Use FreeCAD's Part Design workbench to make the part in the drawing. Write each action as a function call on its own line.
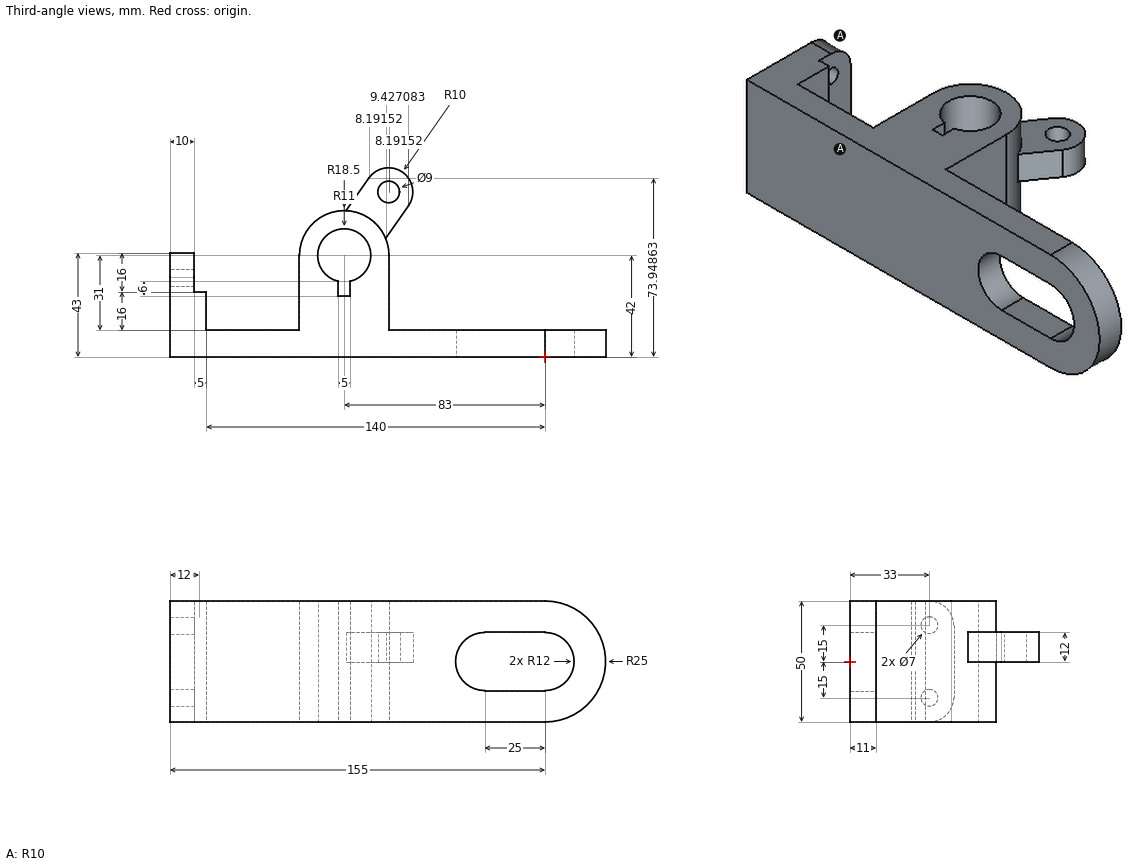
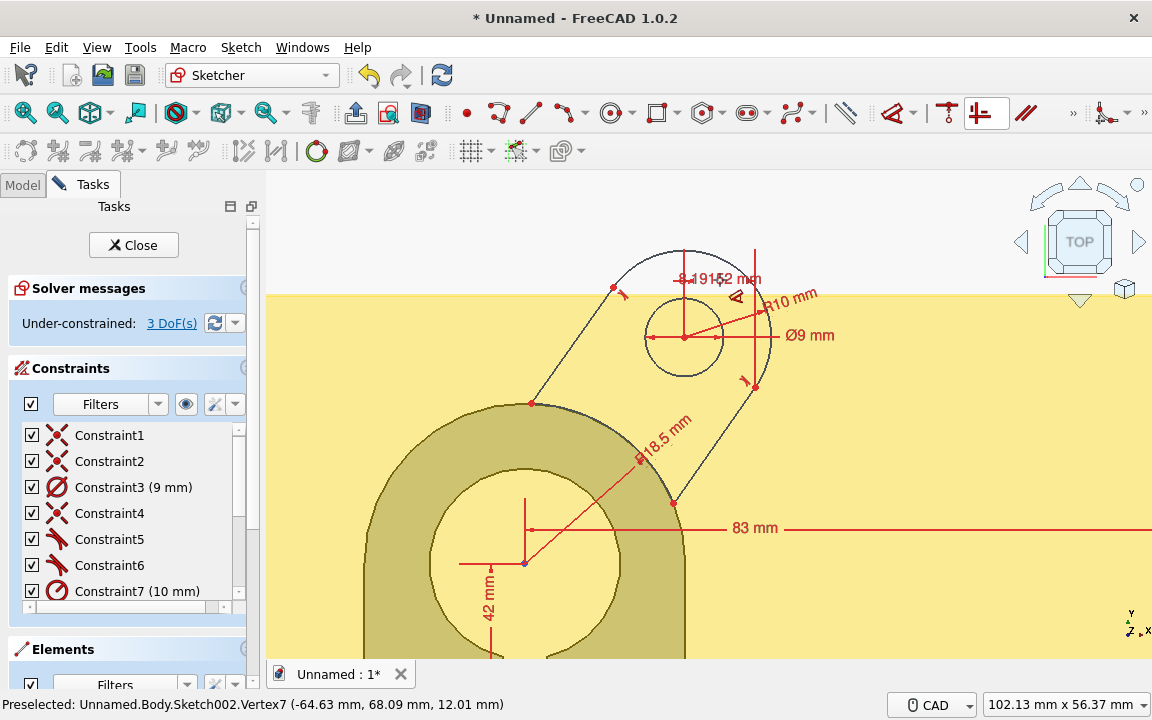
click(614, 287)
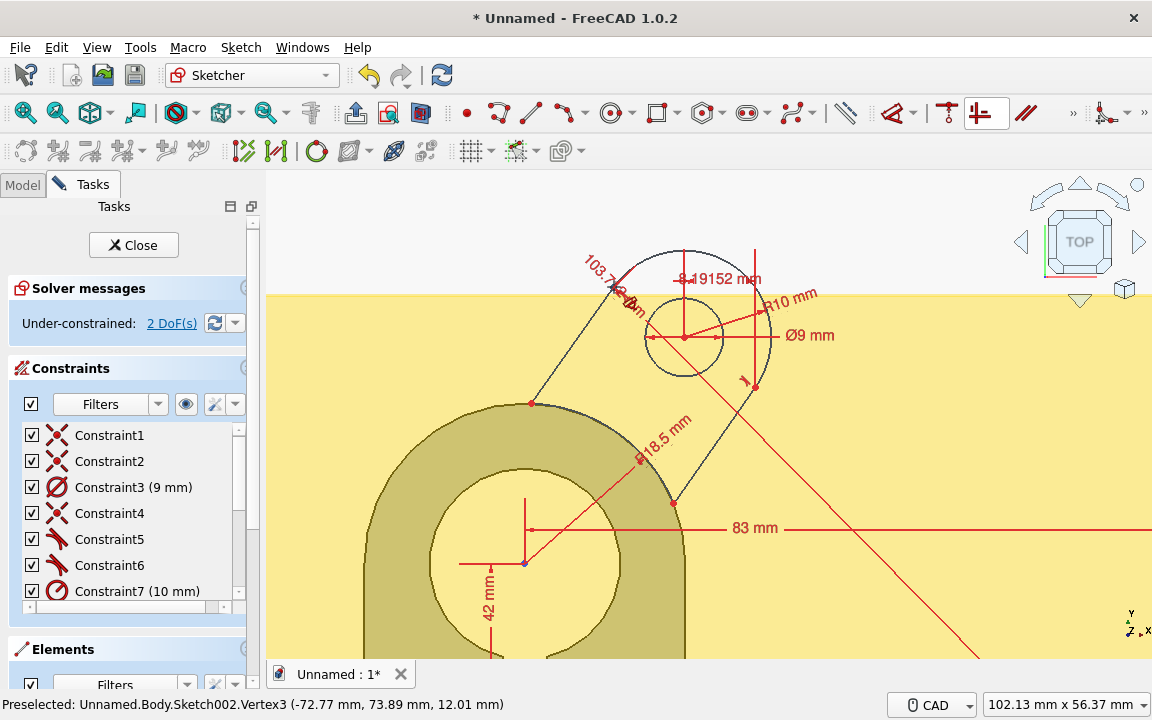
click(684, 337)
click(624, 253)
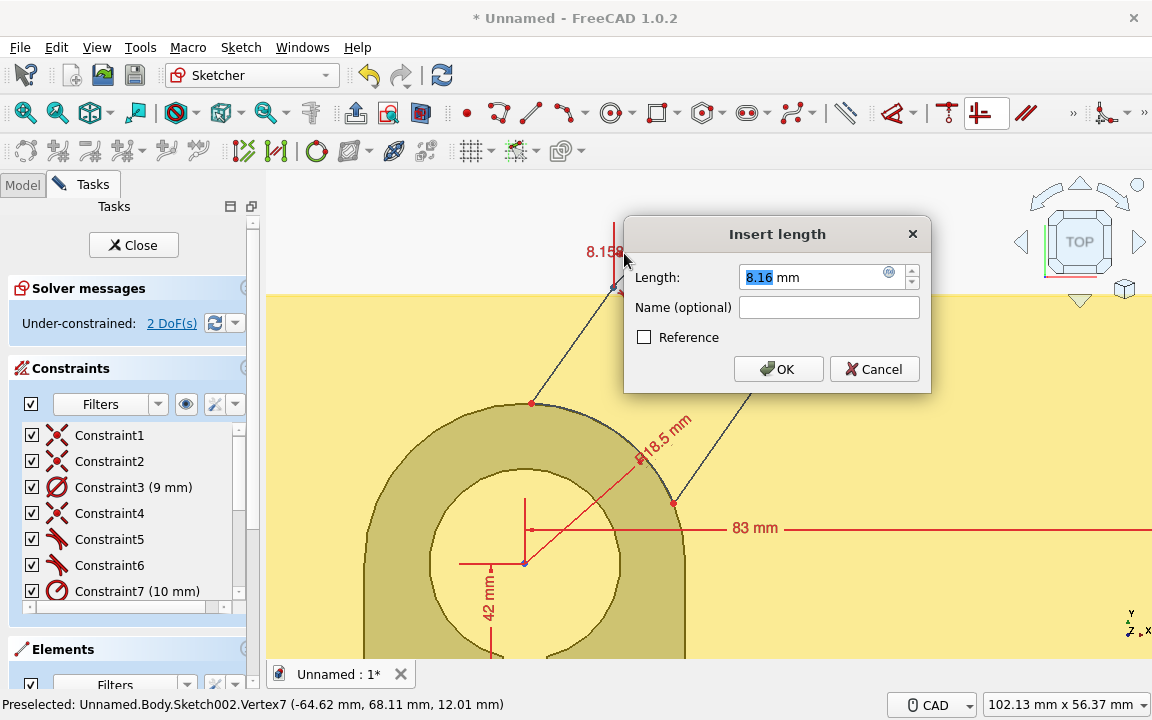
text(8.19152)
key(Return)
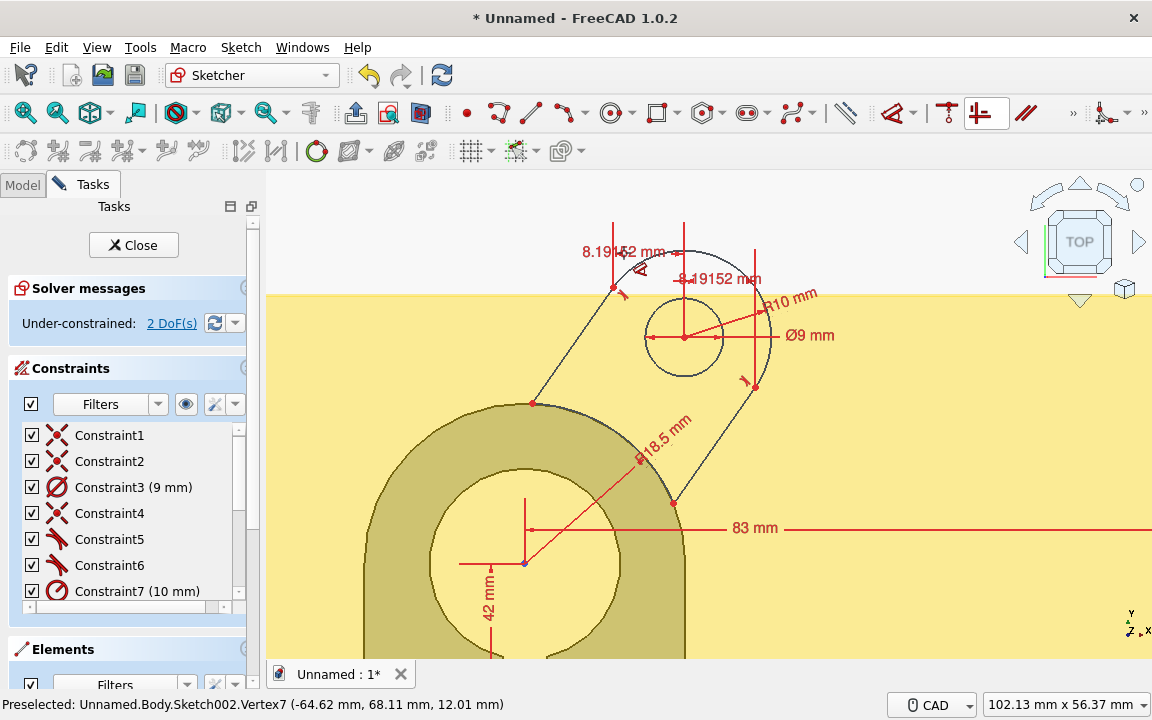
click(613, 288)
click(579, 459)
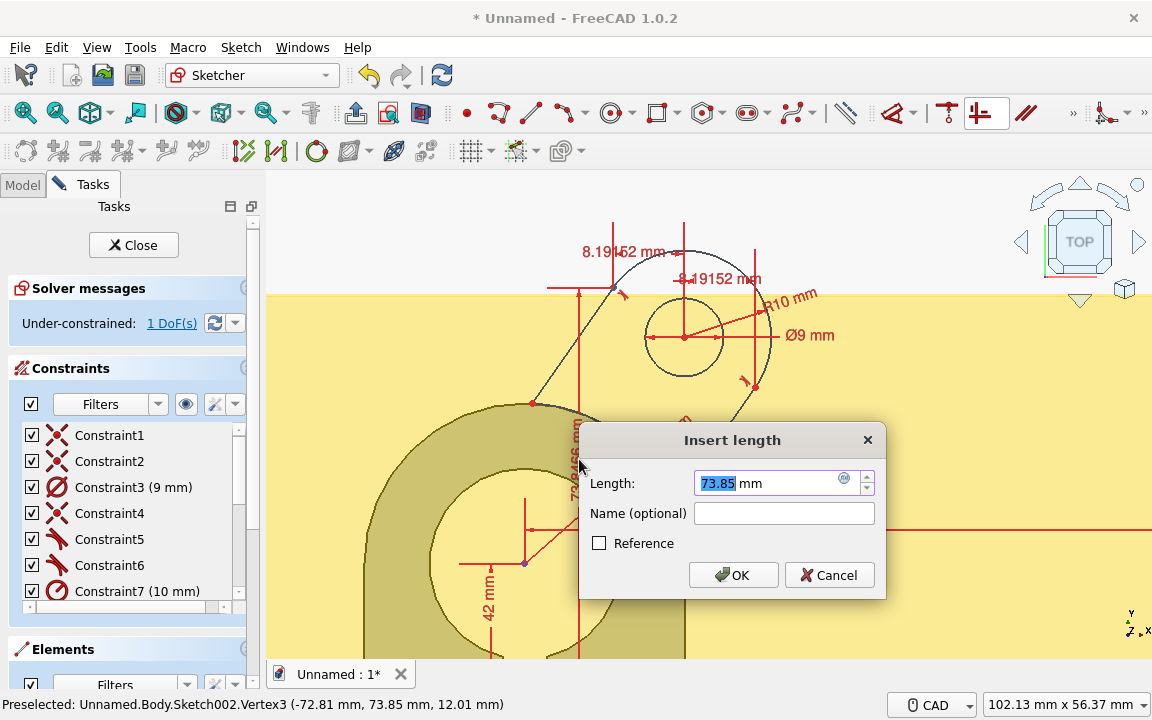
text(73.94863)
key(Return)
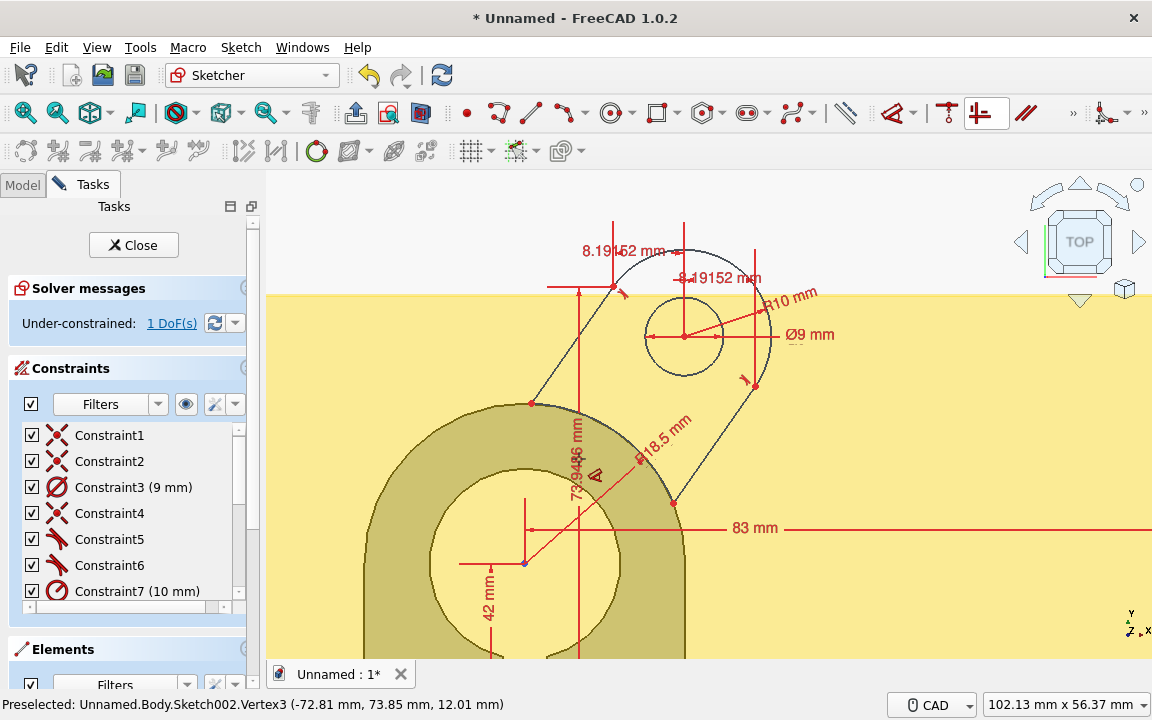
click(698, 468)
click(686, 537)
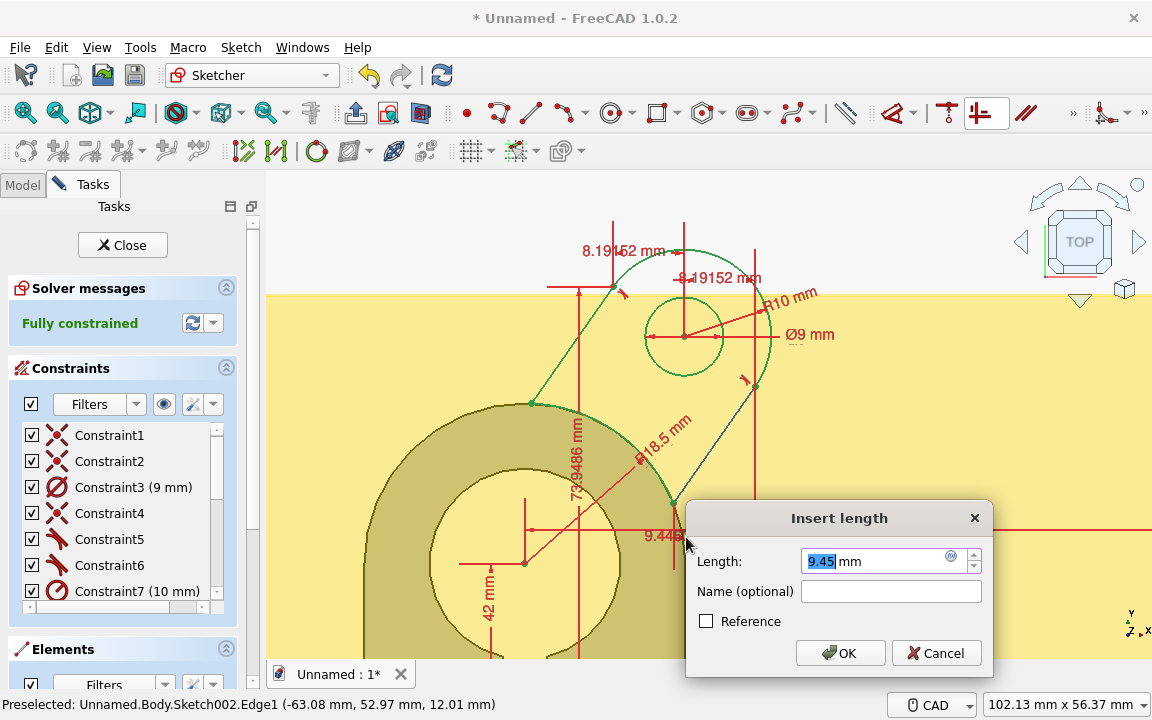
text(9.427083)
key(Return)
key(Escape)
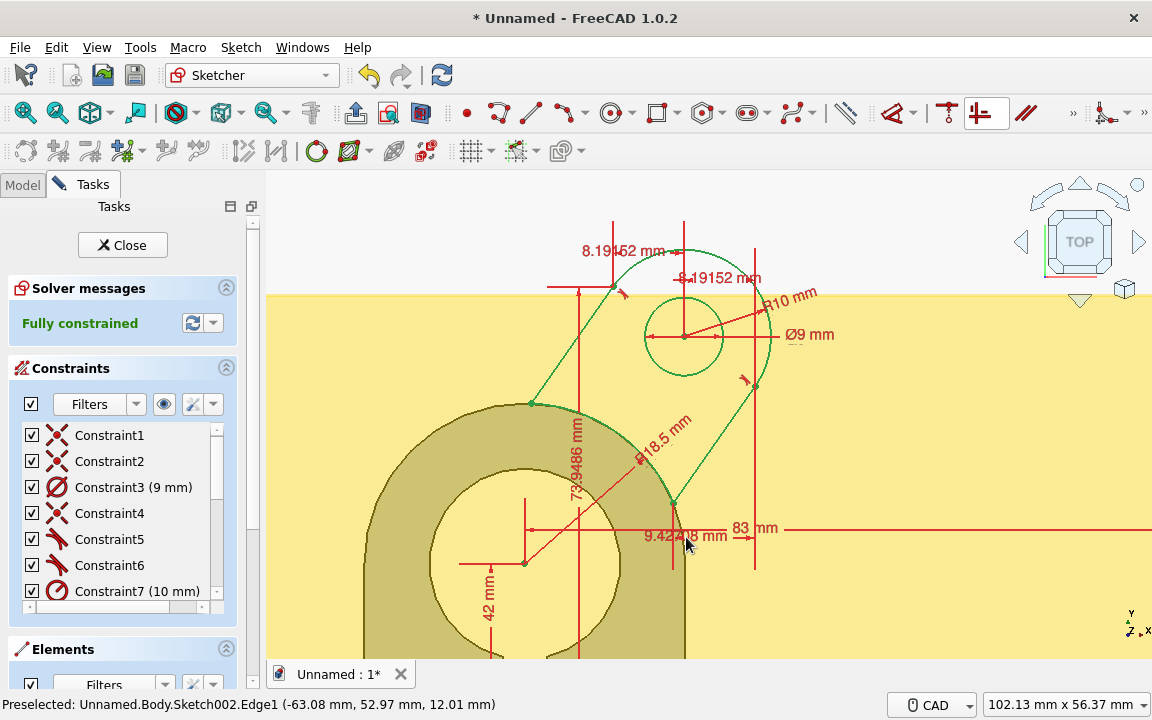
click(123, 245)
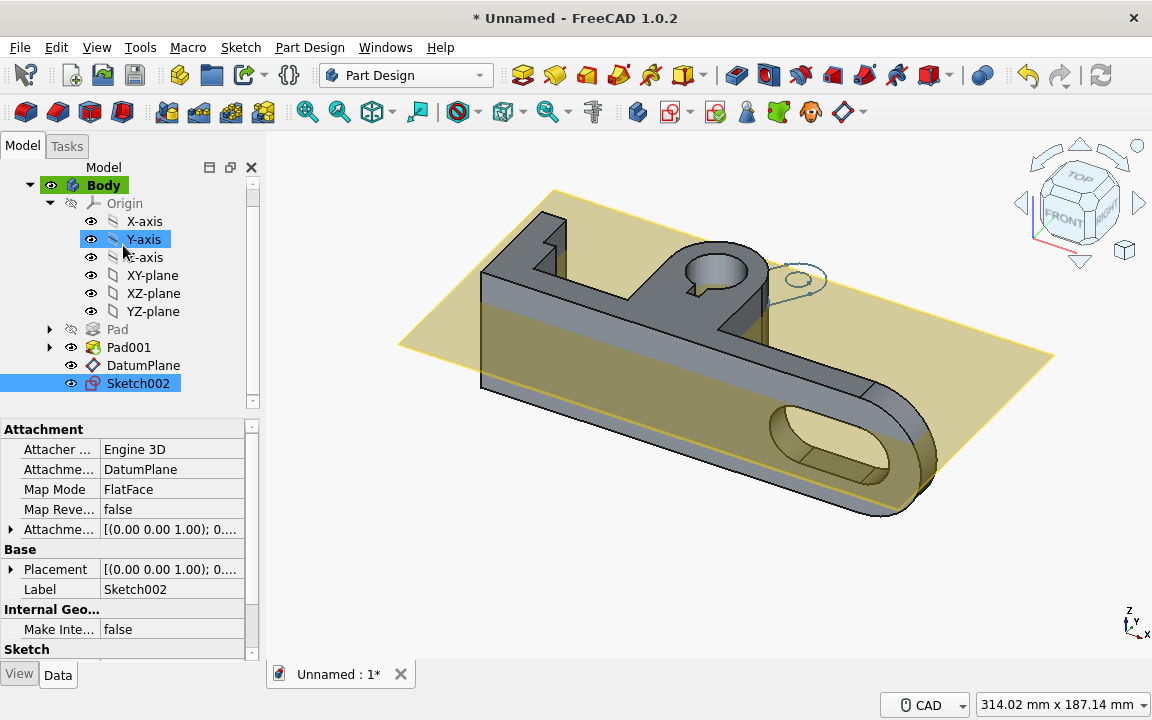
click(524, 76)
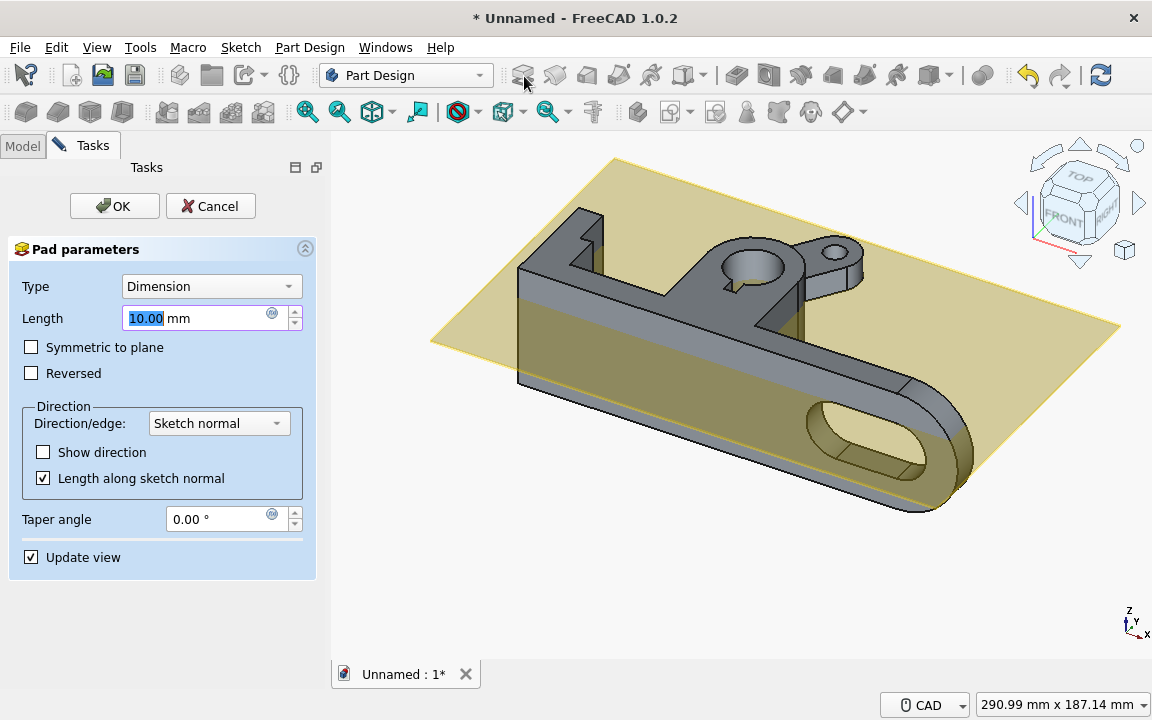
text(12)
key(Tab)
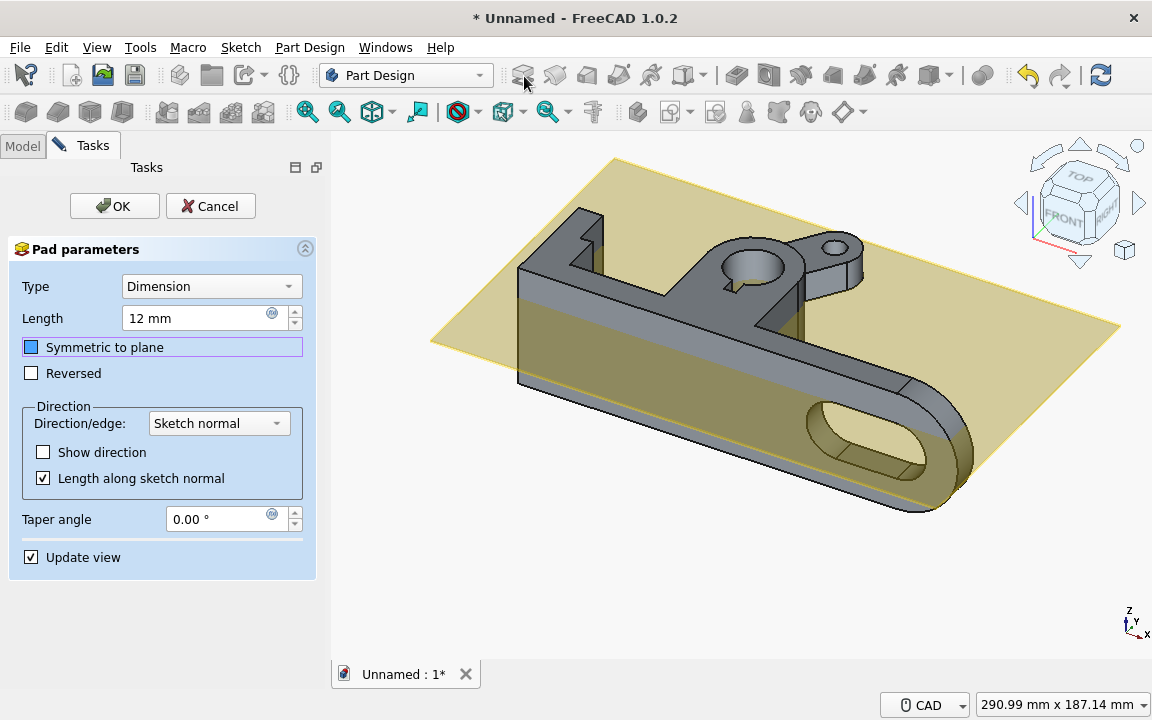
click(30, 373)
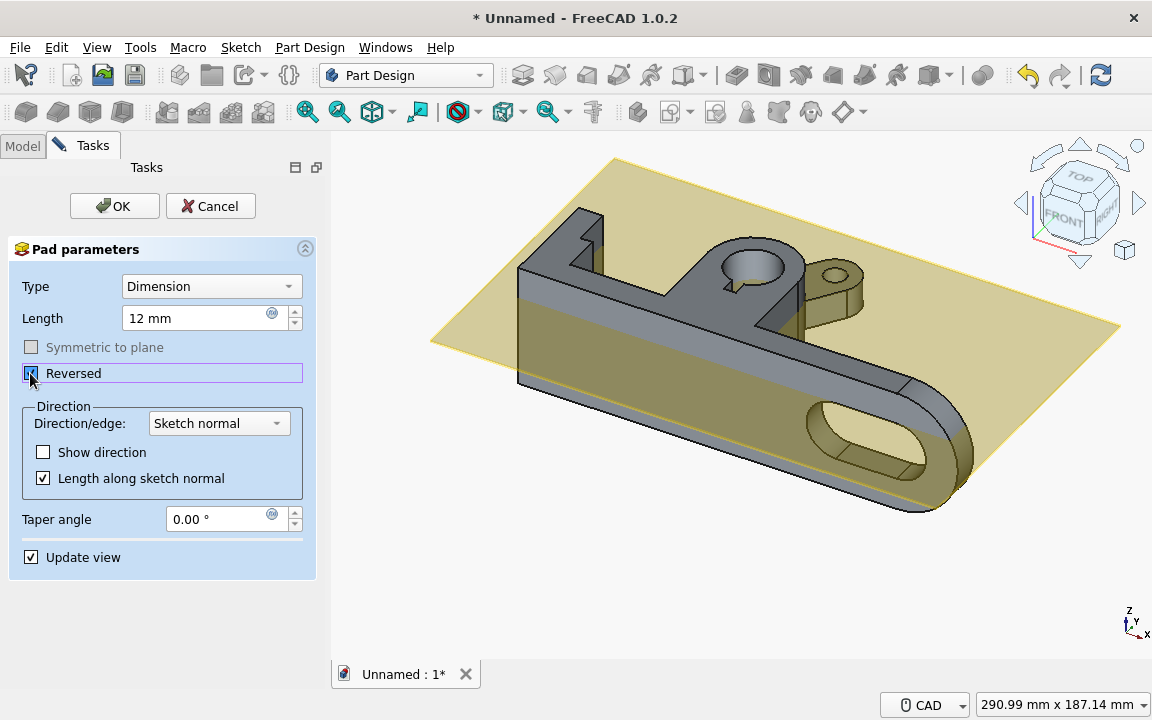
click(115, 206)